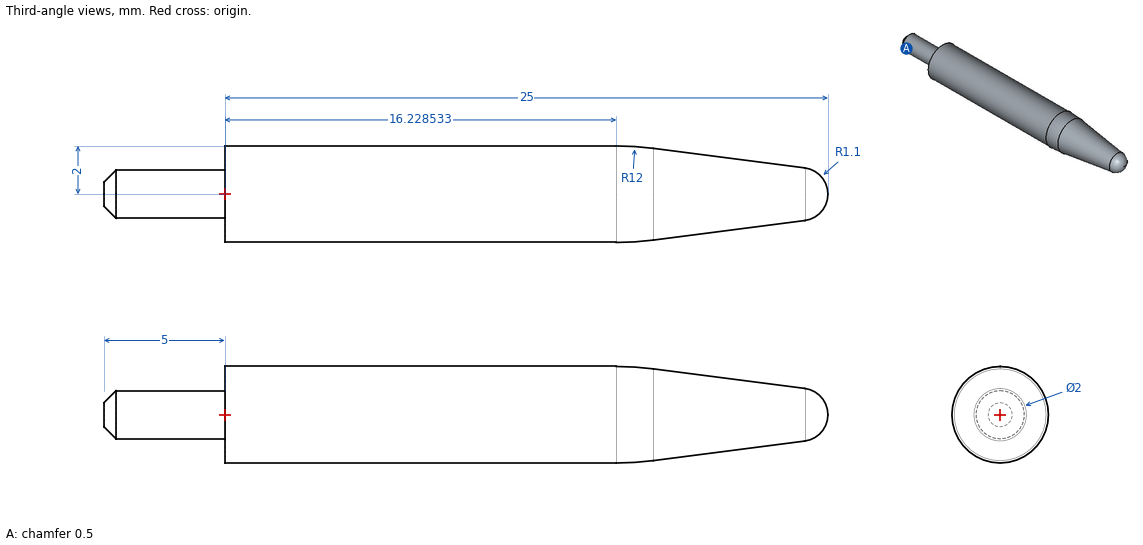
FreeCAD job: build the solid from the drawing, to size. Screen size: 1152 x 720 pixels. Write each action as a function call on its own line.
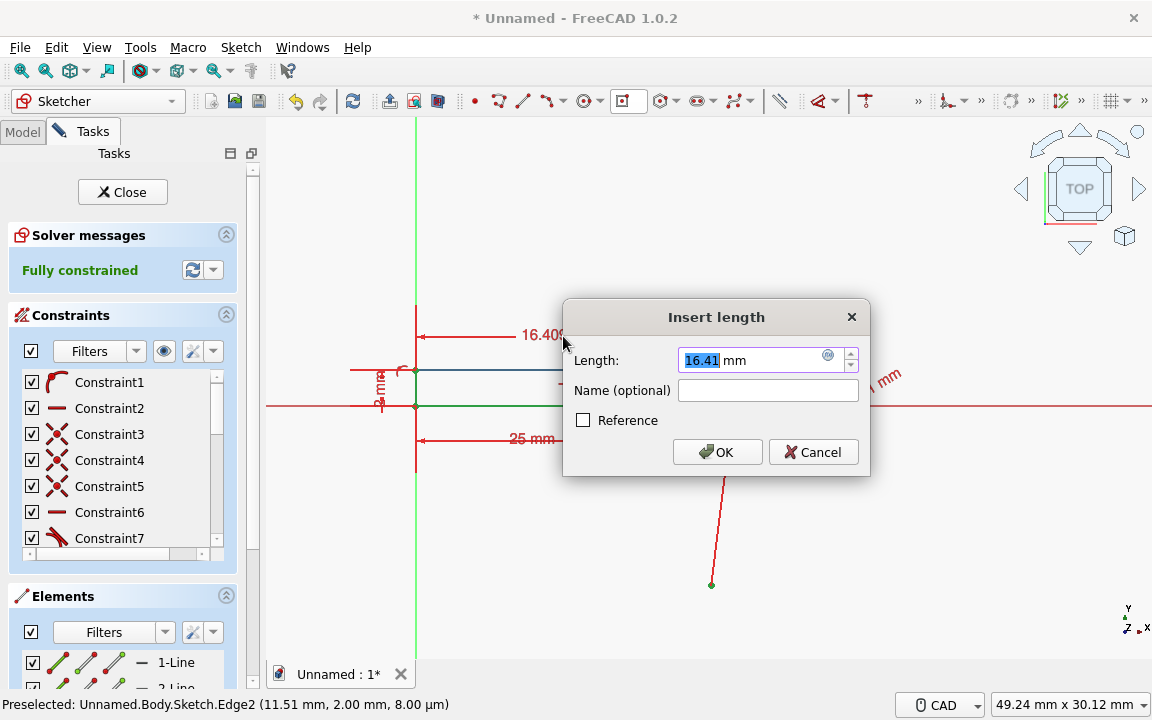
text(16.228533)
key(Return)
key(Escape)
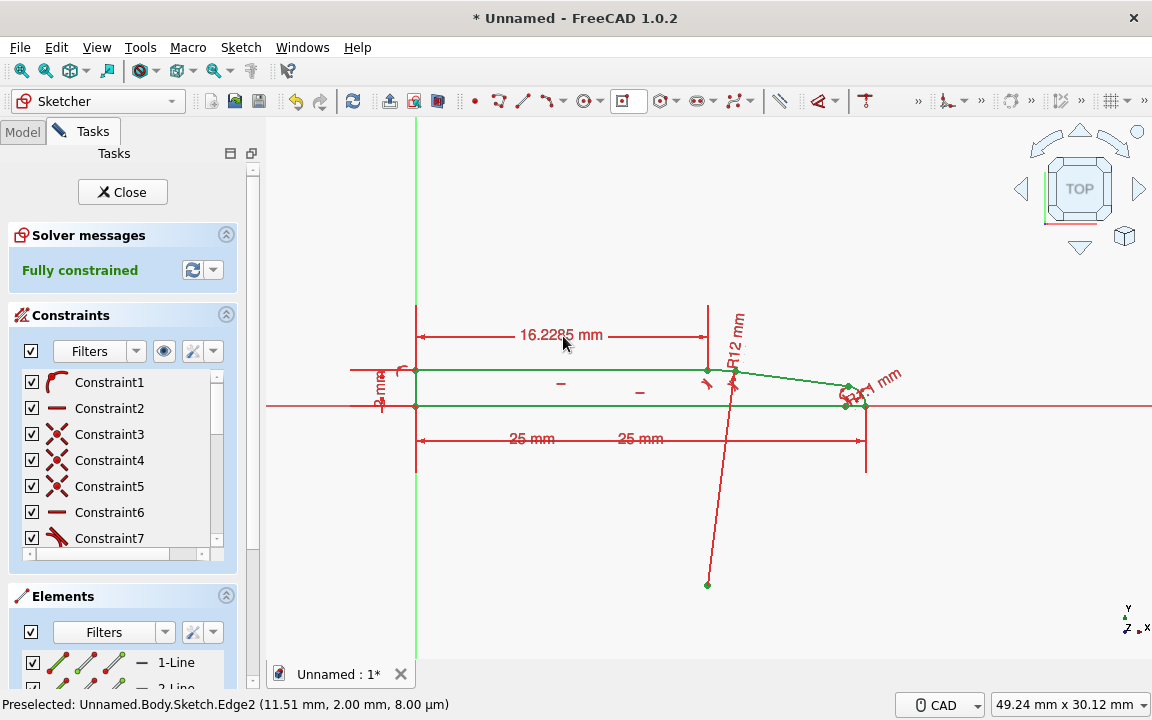
click(123, 192)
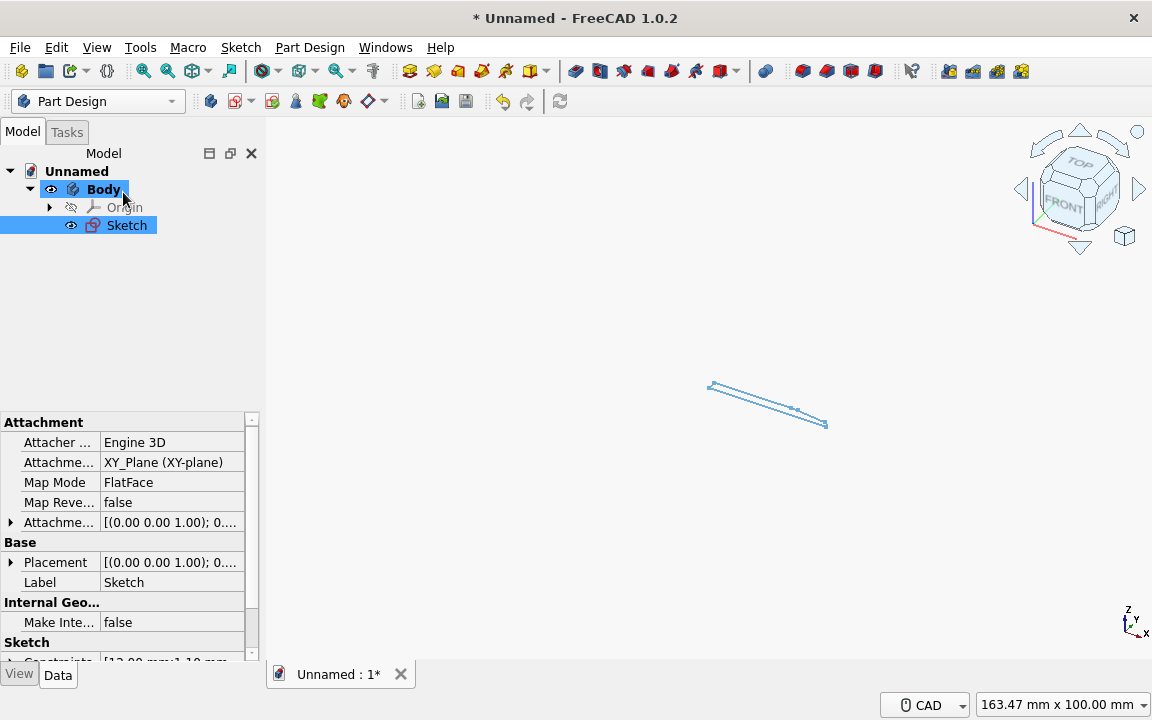
click(434, 72)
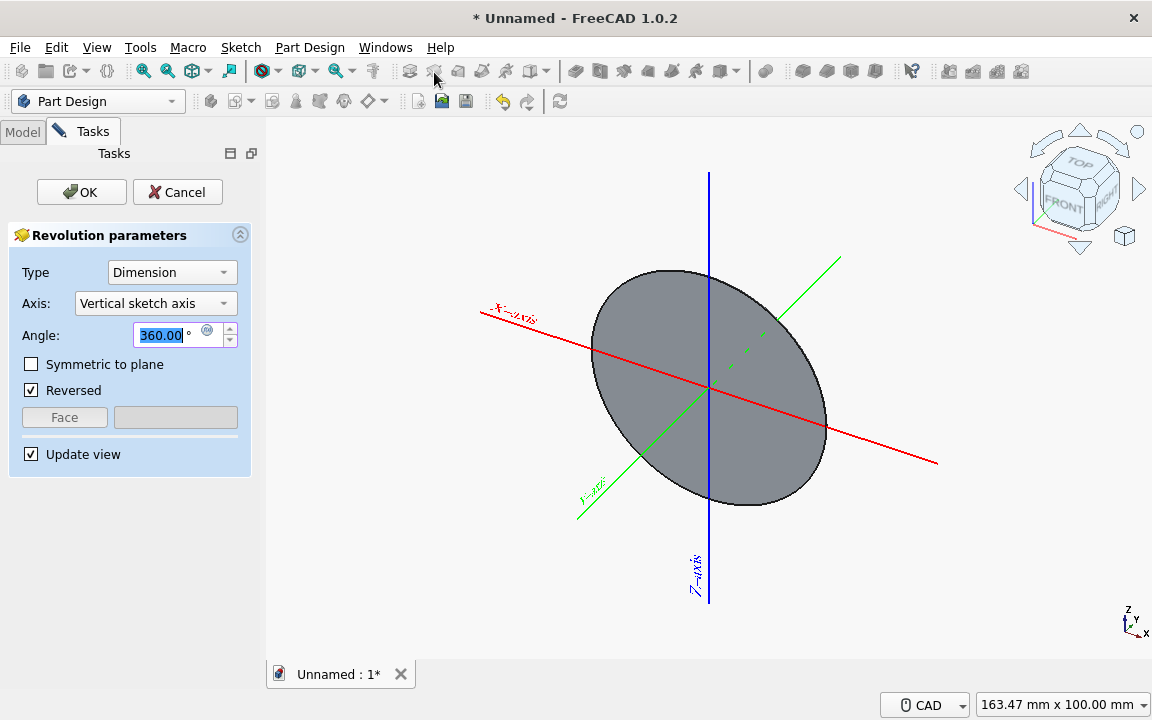
click(156, 304)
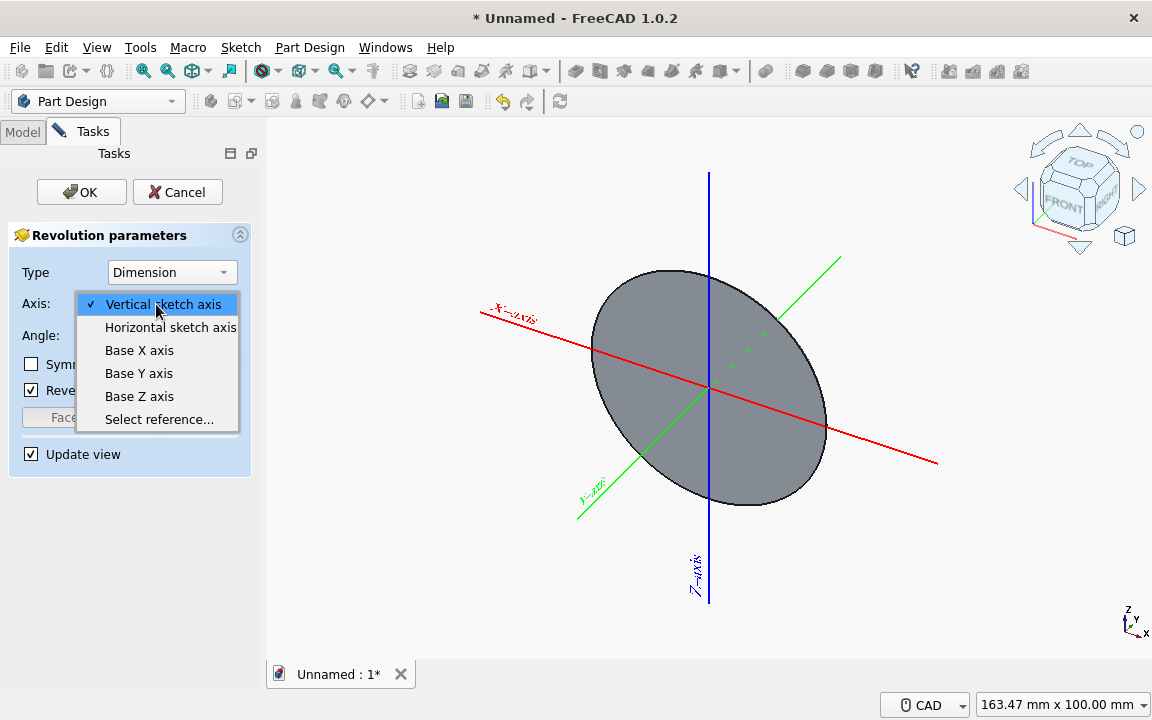
click(156, 328)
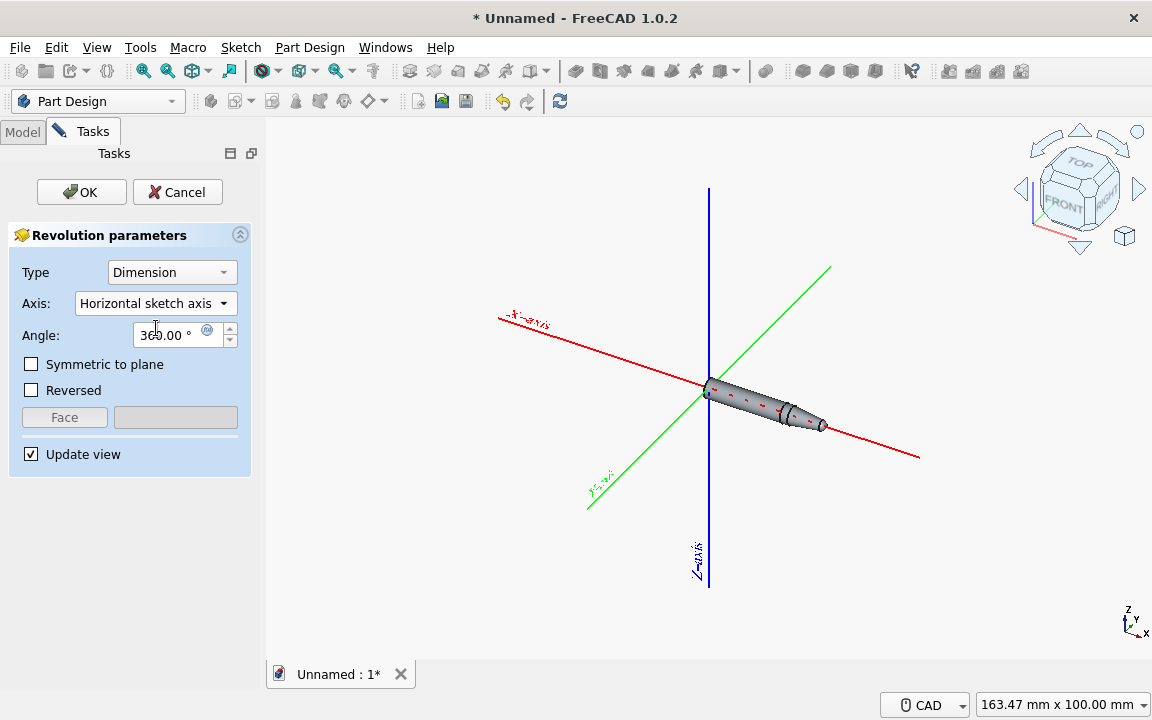
click(82, 192)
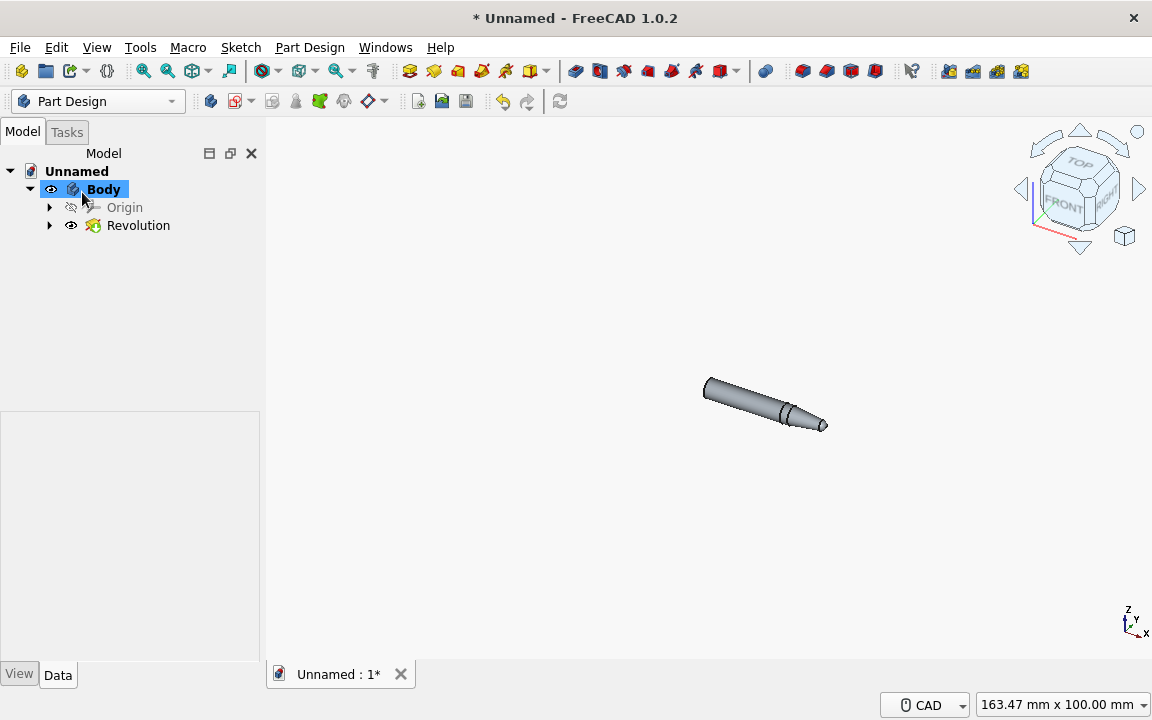
key(v)
key(f)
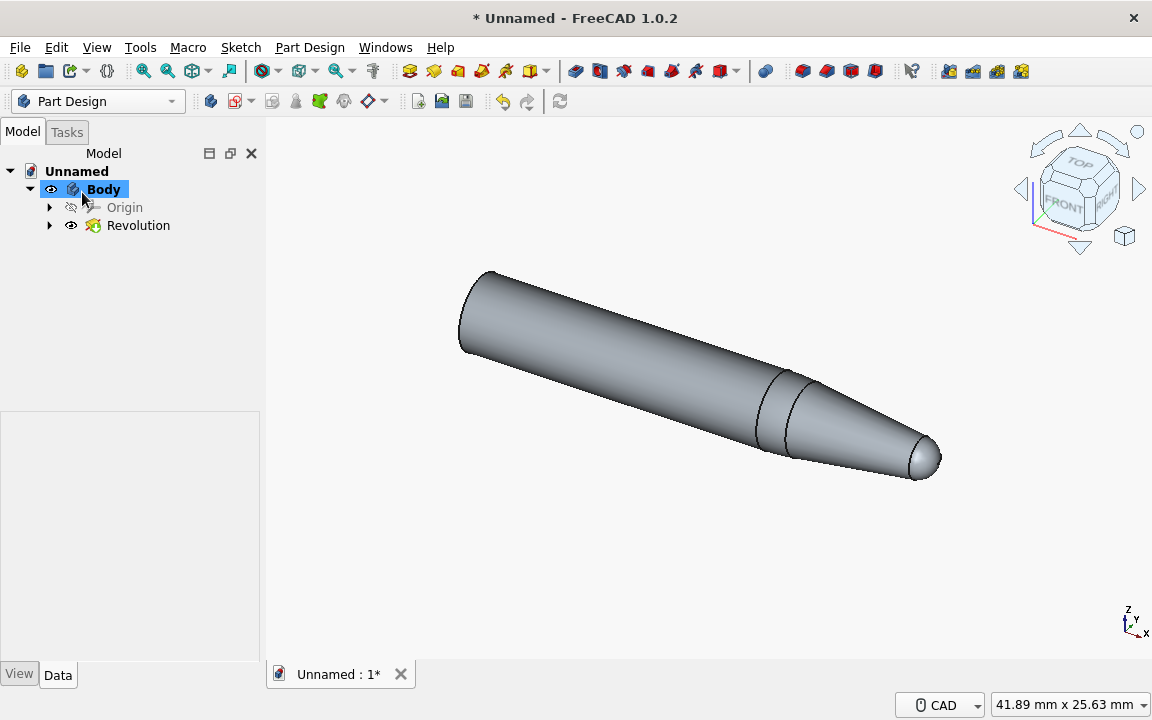
click(236, 102)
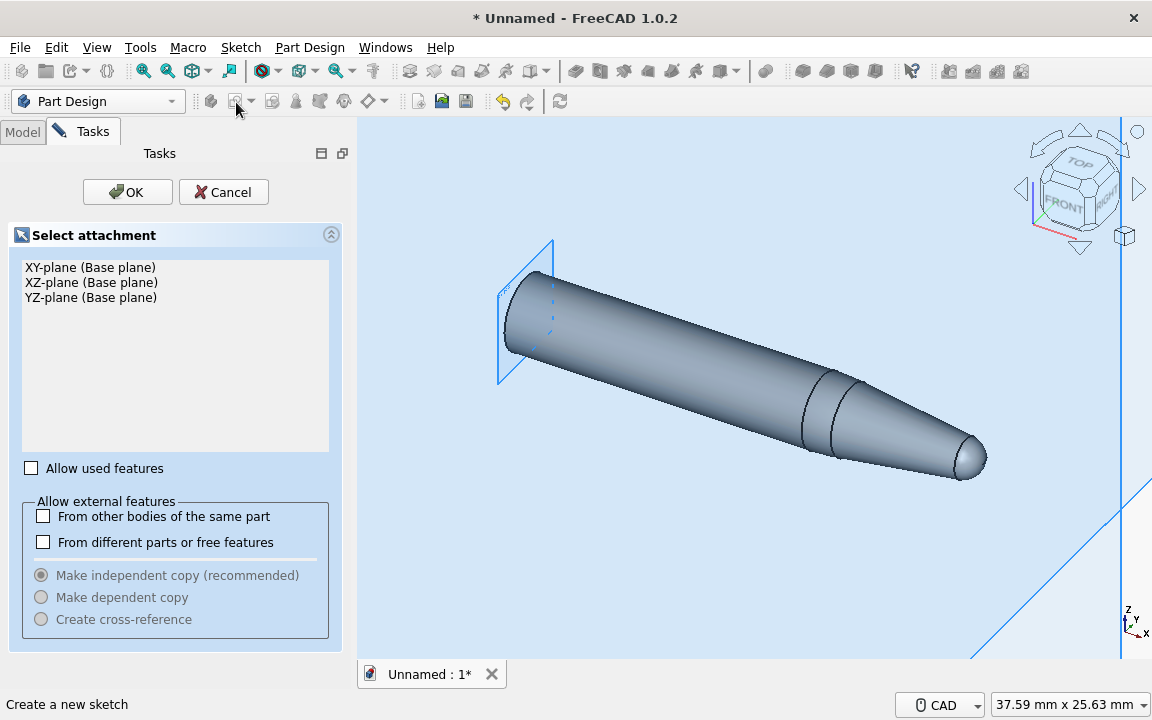
click(82, 298)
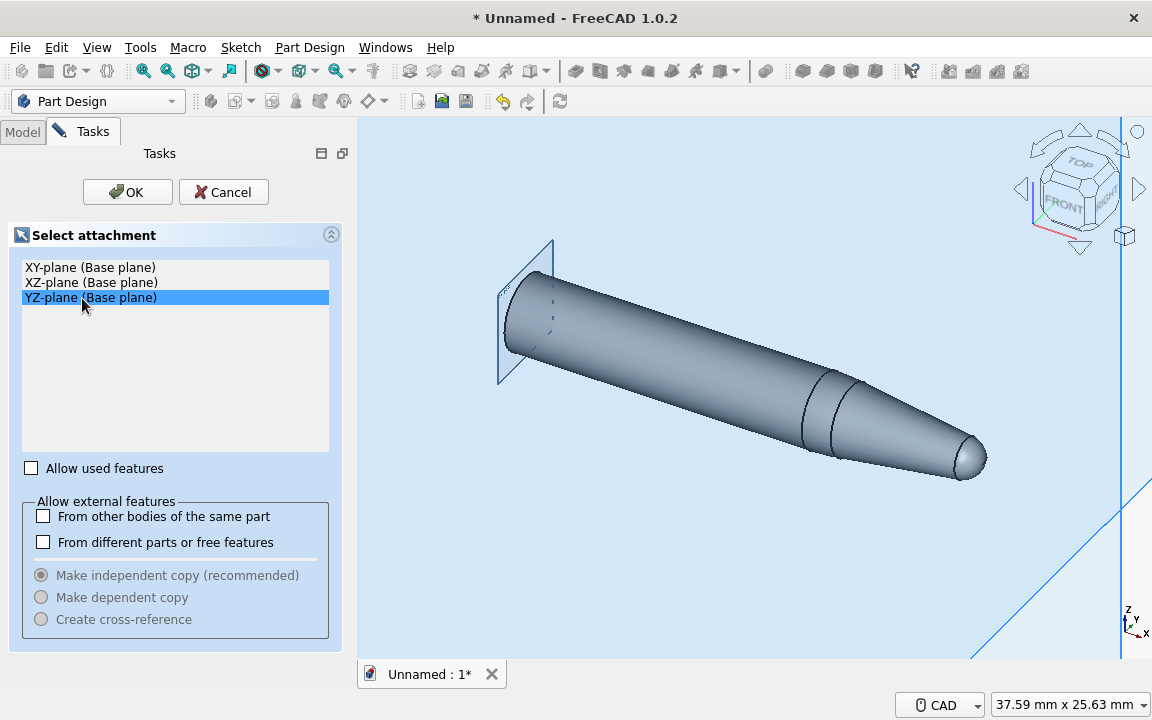
click(128, 192)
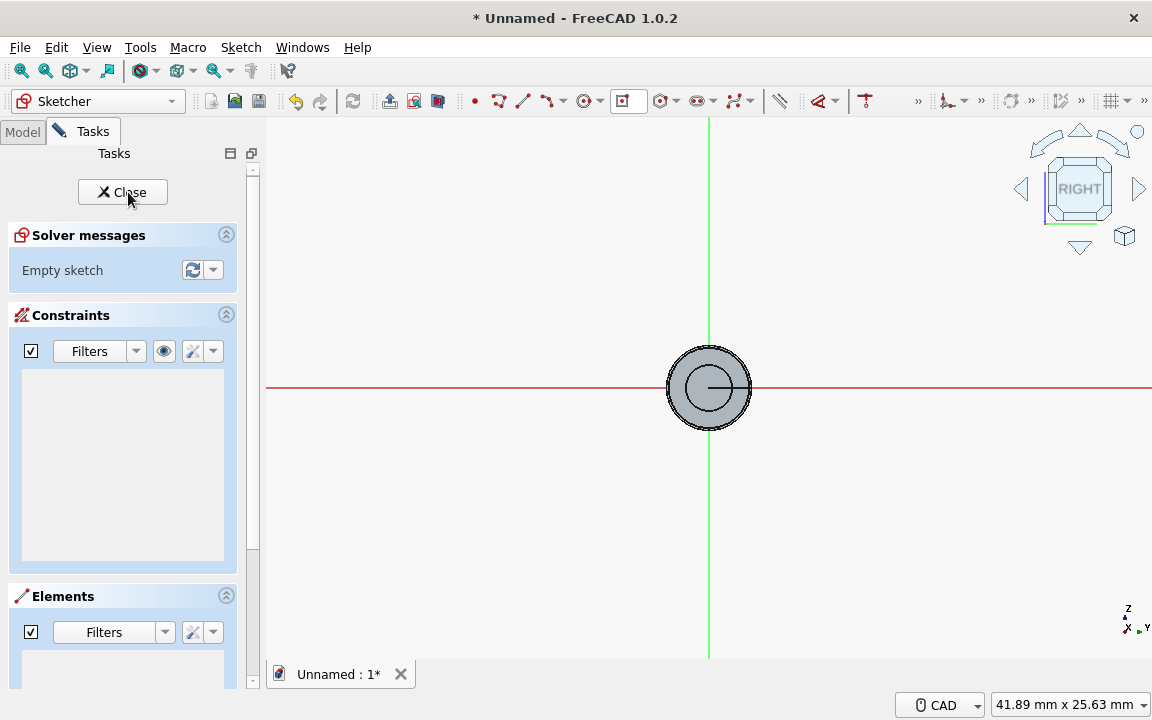
click(438, 102)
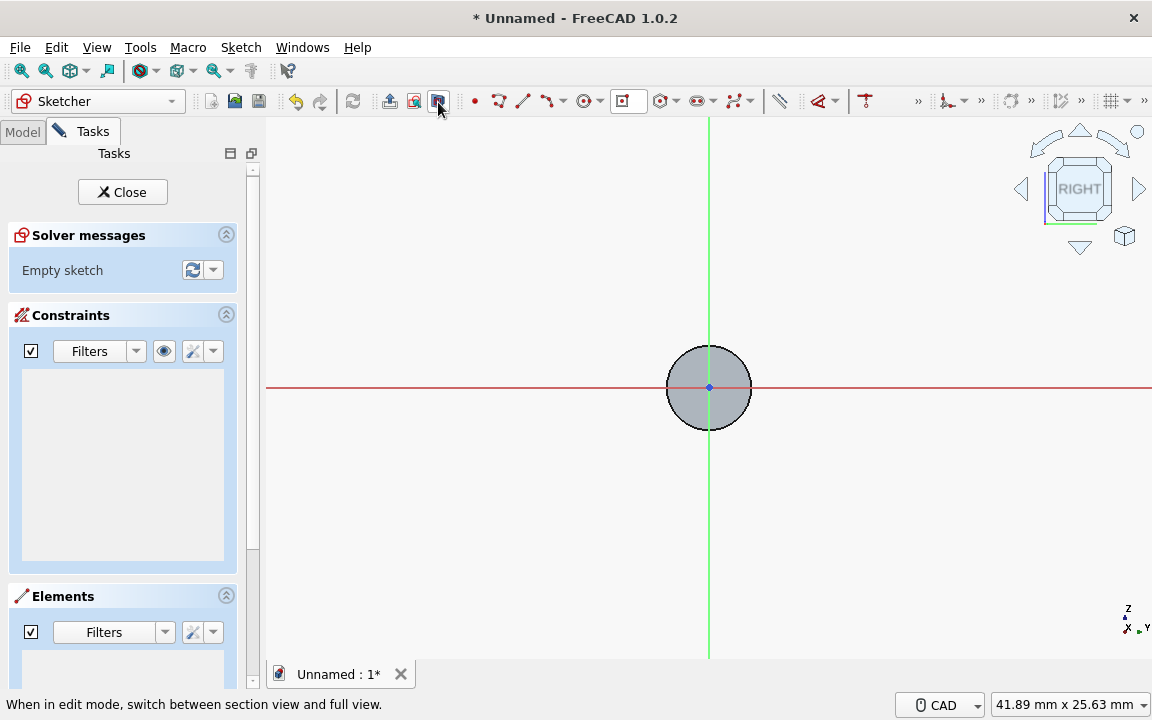
scroll(720, 388, up, 10)